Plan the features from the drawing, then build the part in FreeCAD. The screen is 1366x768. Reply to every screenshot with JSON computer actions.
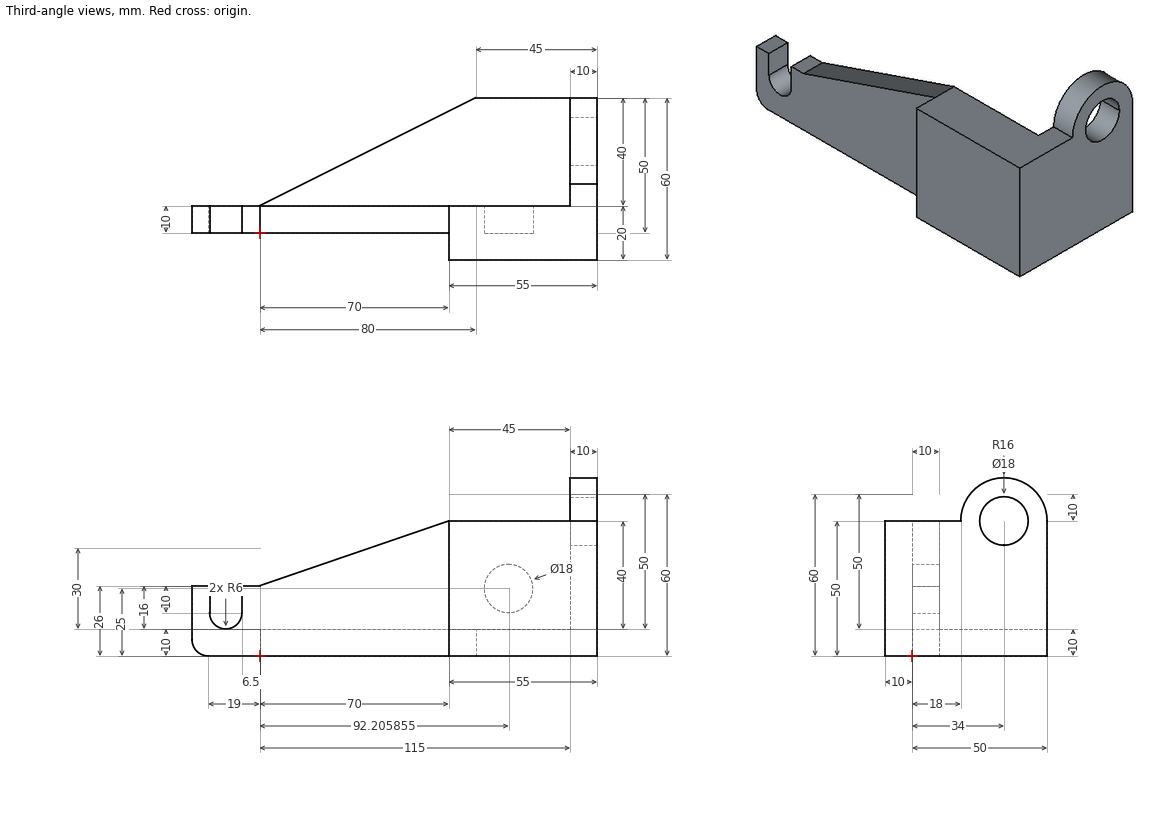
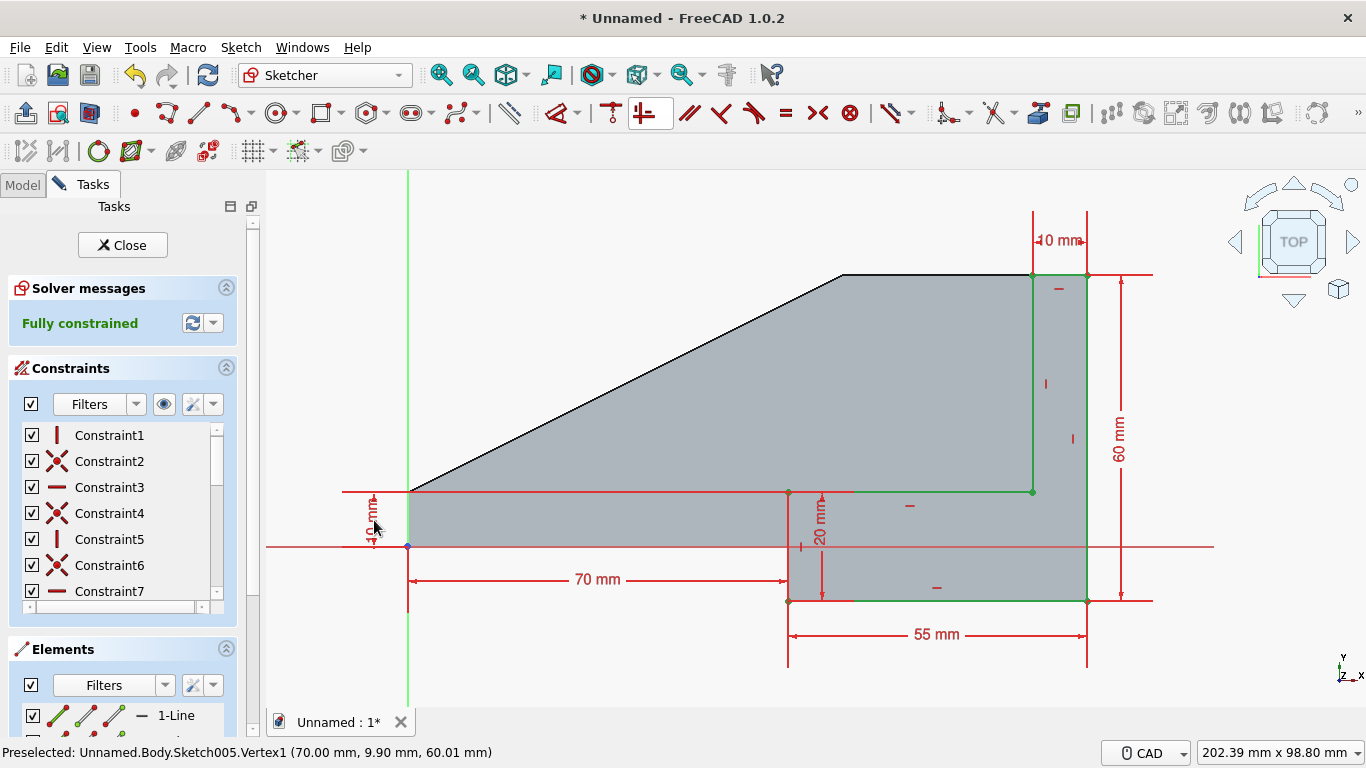
{"action": "left_click", "coordinate": [123, 245]}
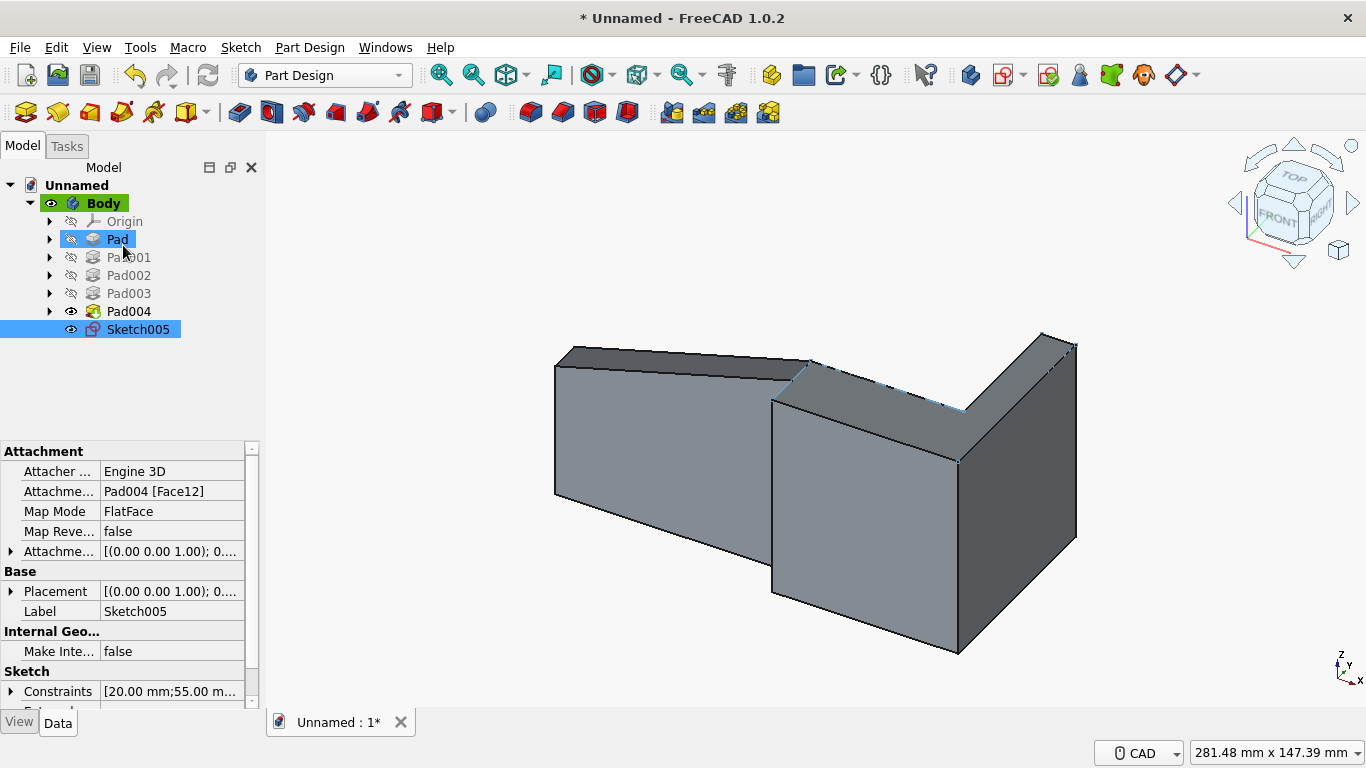
{"action": "left_click", "coordinate": [240, 112]}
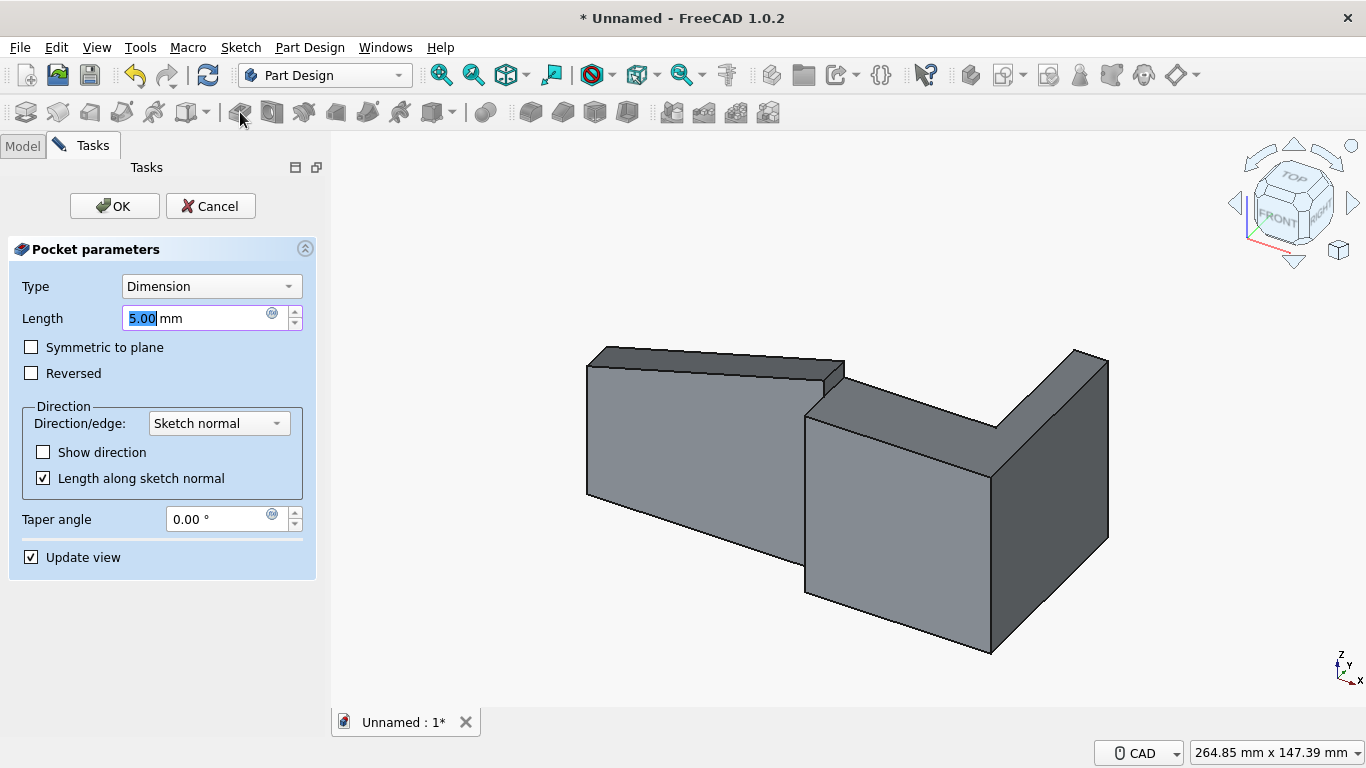
{"action": "type", "text": "10"}
{"action": "key", "text": "Tab"}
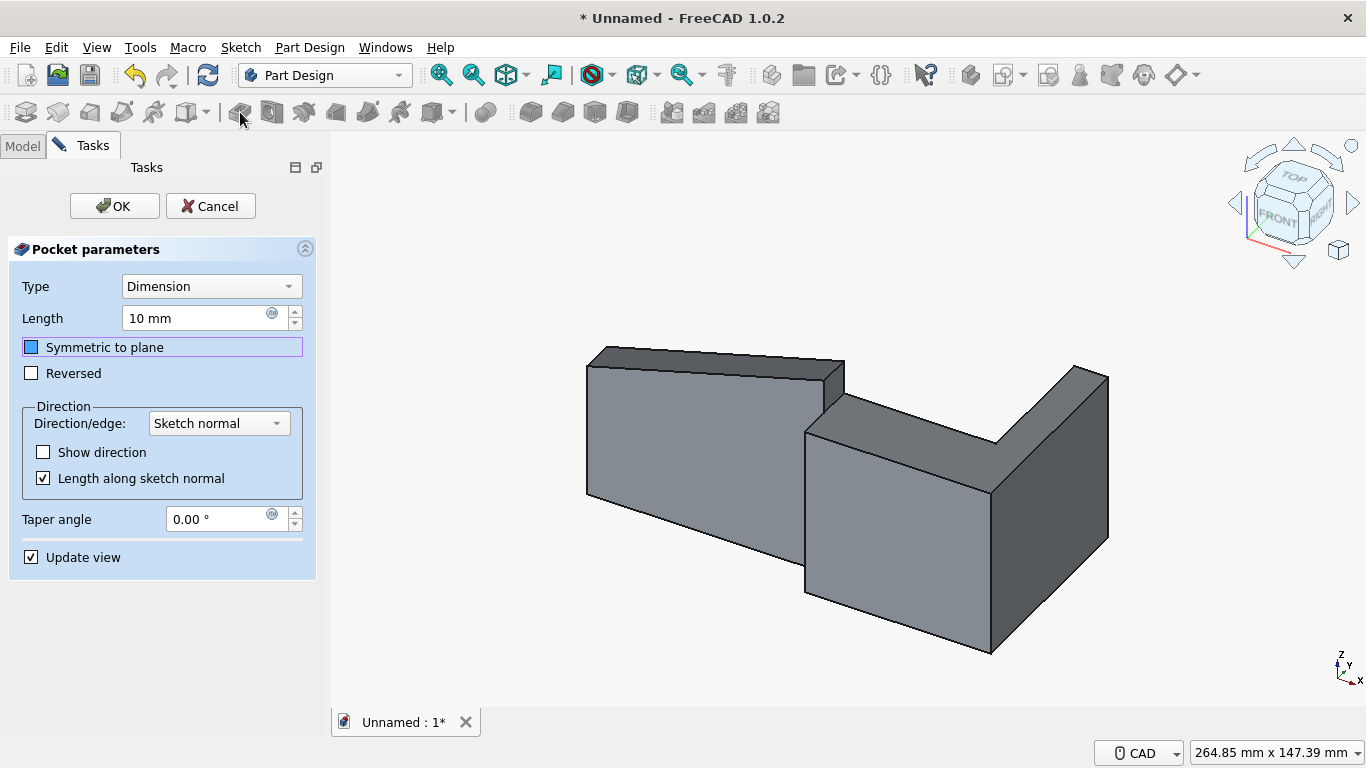
{"action": "left_click", "coordinate": [115, 206]}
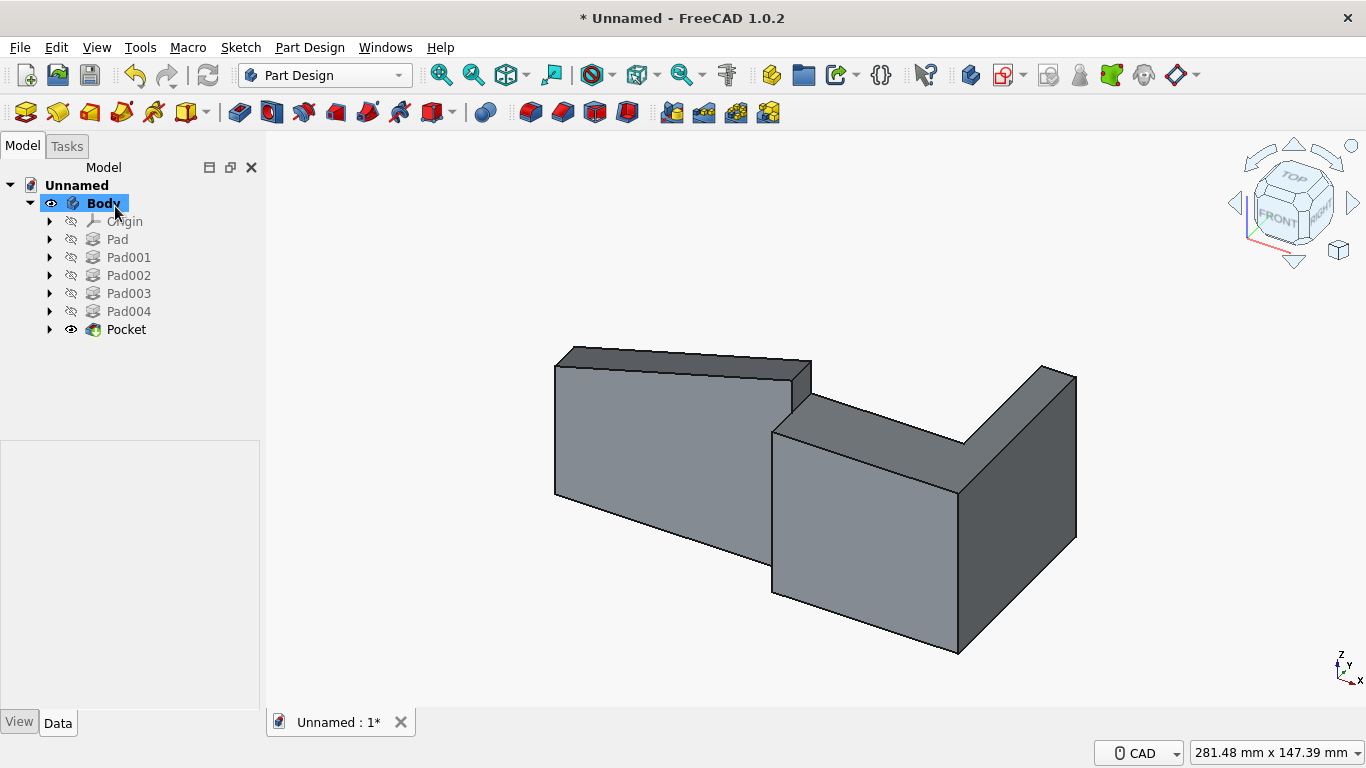
{"action": "key", "text": "4"}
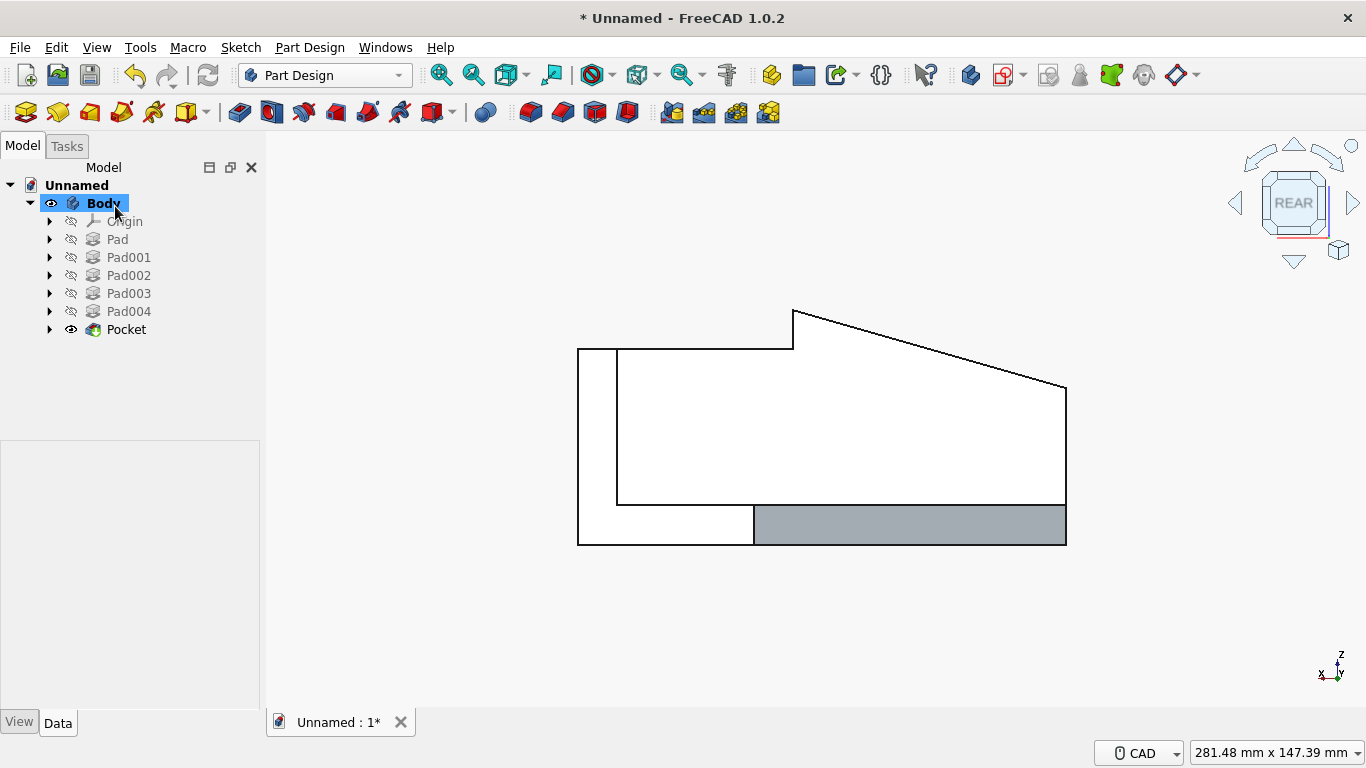
{"action": "left_click", "coordinate": [442, 76]}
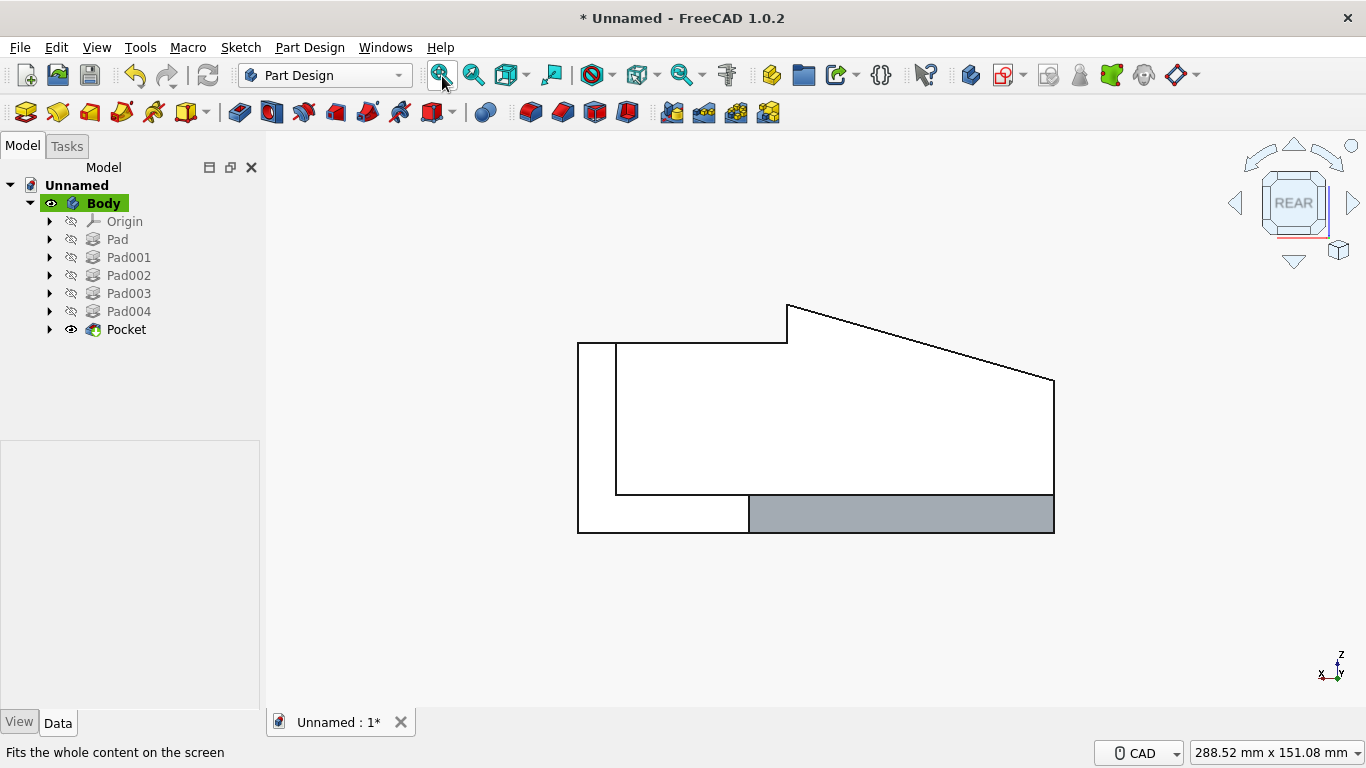
{"action": "left_click", "coordinate": [835, 399]}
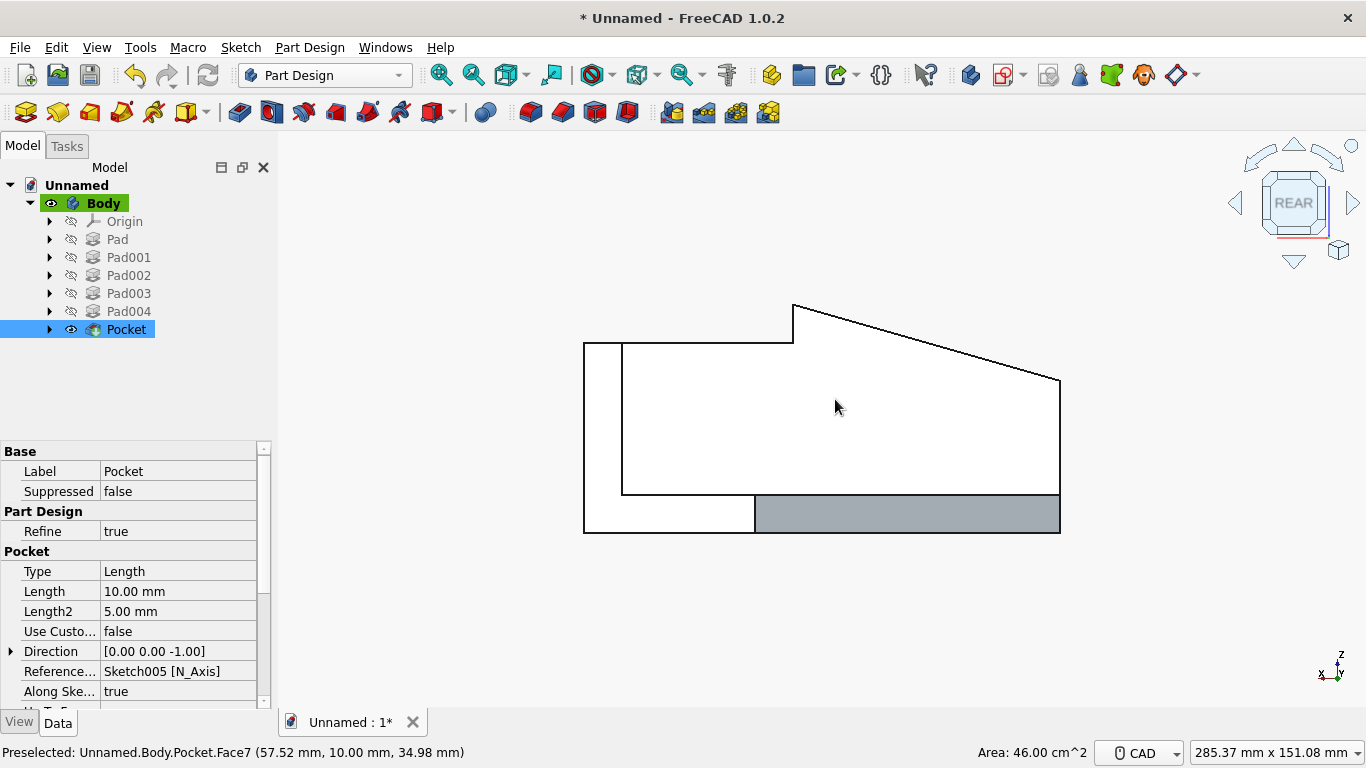
{"action": "left_click", "coordinate": [1004, 76]}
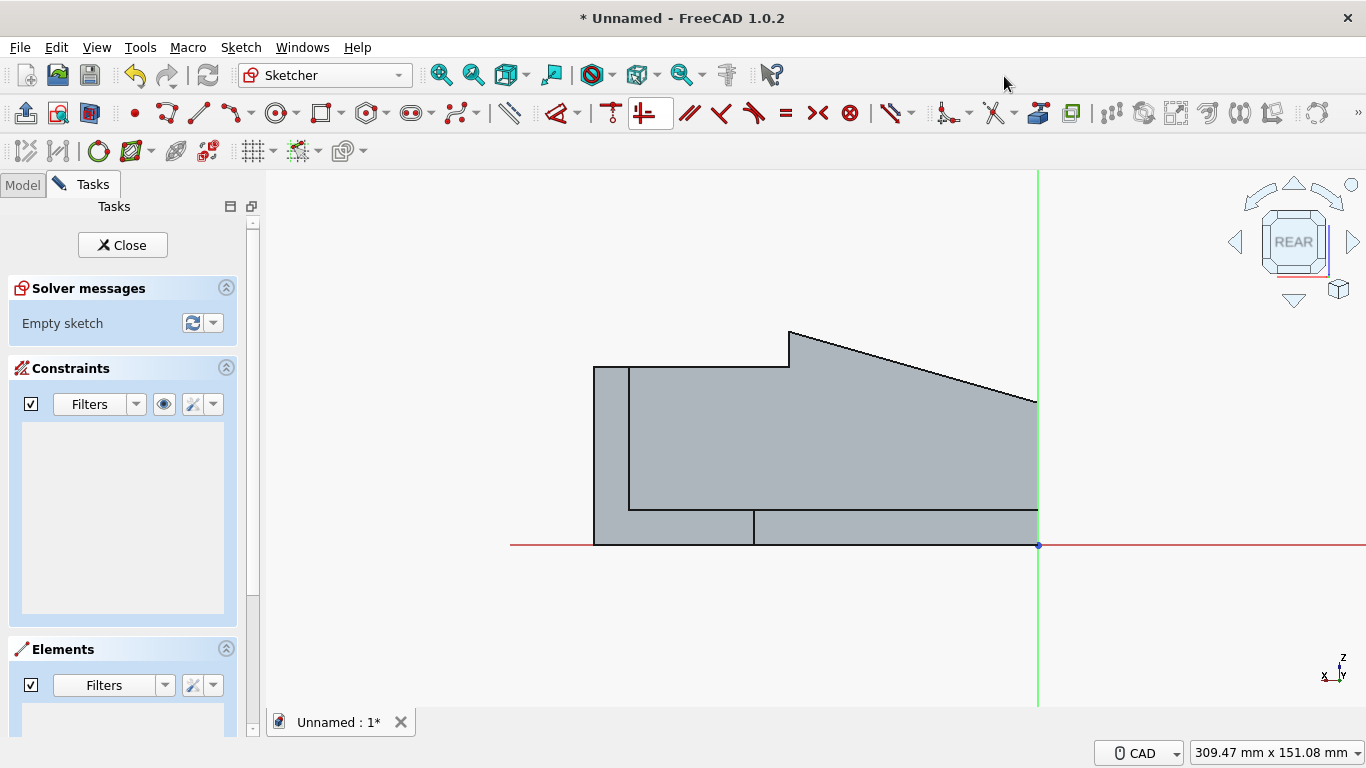
{"action": "scroll", "coordinate": [1201, 439], "scroll_direction": "up", "scroll_amount": 2}